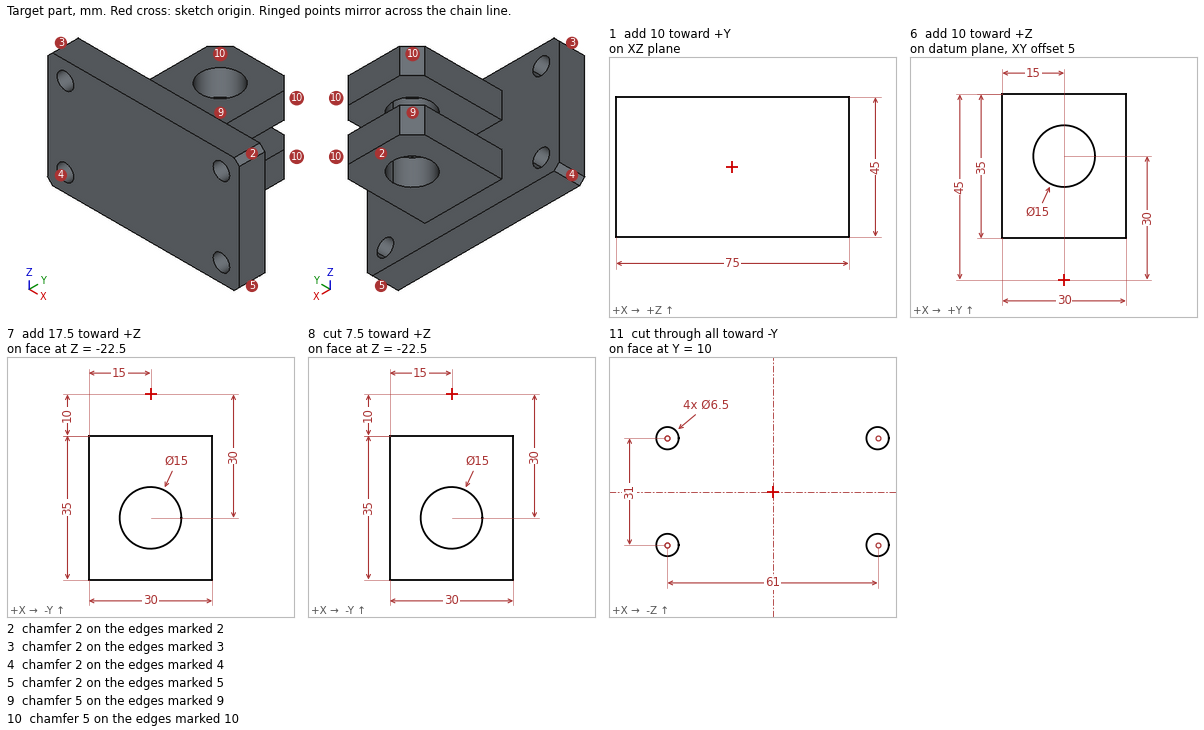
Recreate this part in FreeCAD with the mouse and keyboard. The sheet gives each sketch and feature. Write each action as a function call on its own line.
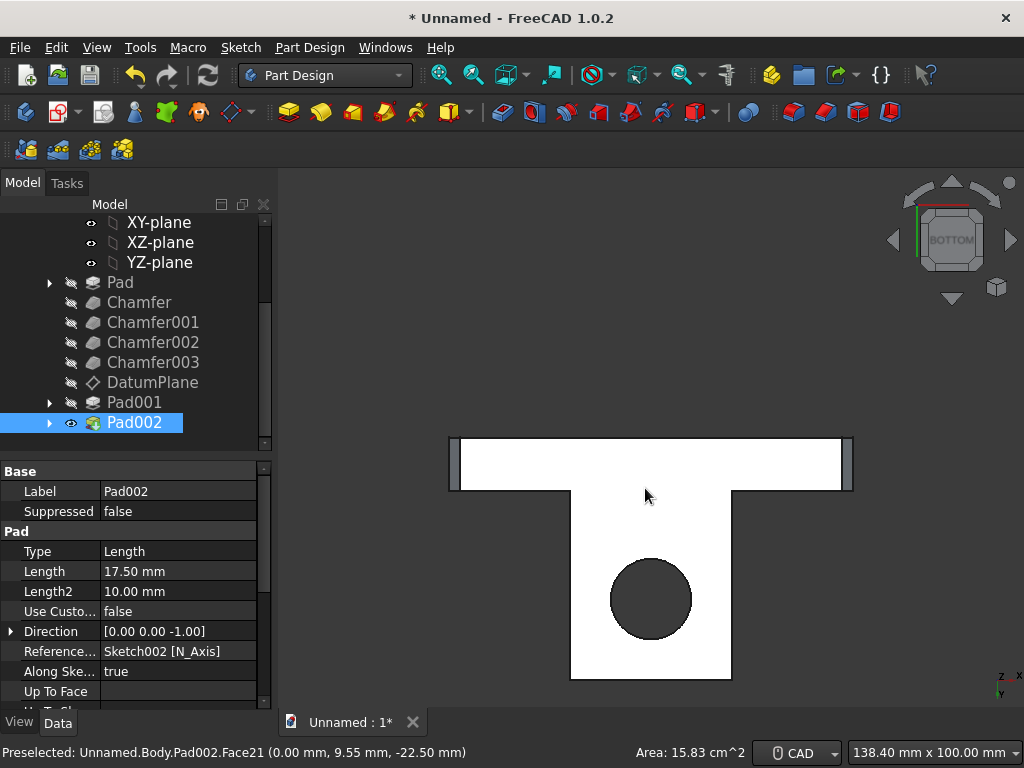
click(58, 112)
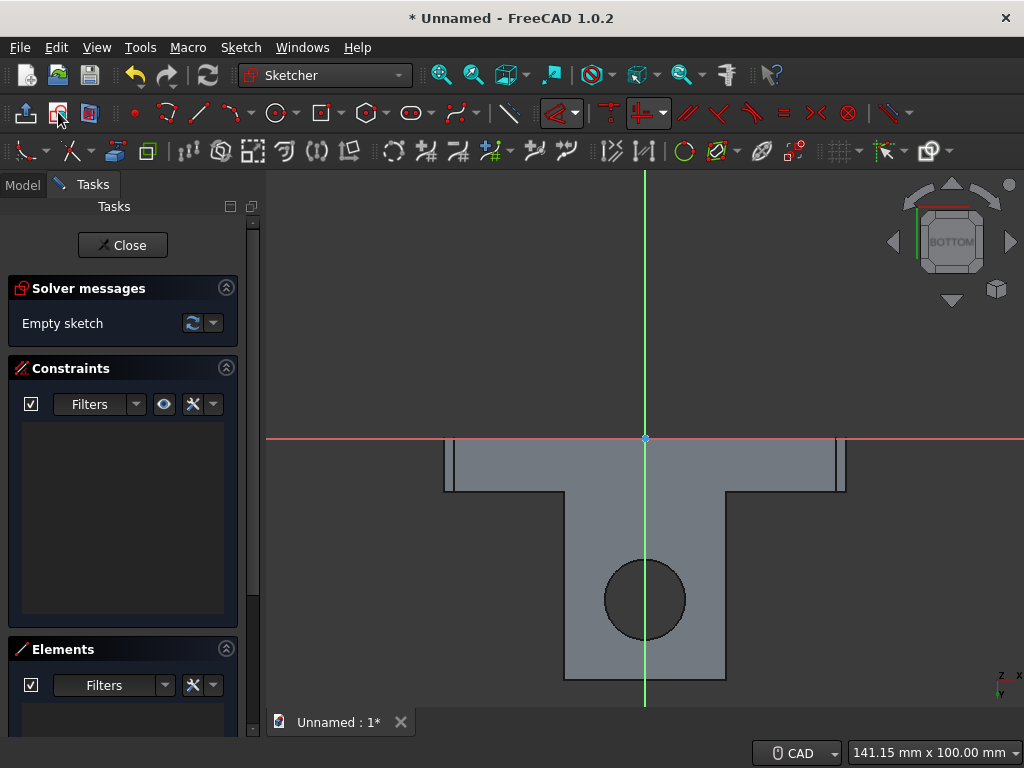
scroll(294, 198, down, 1)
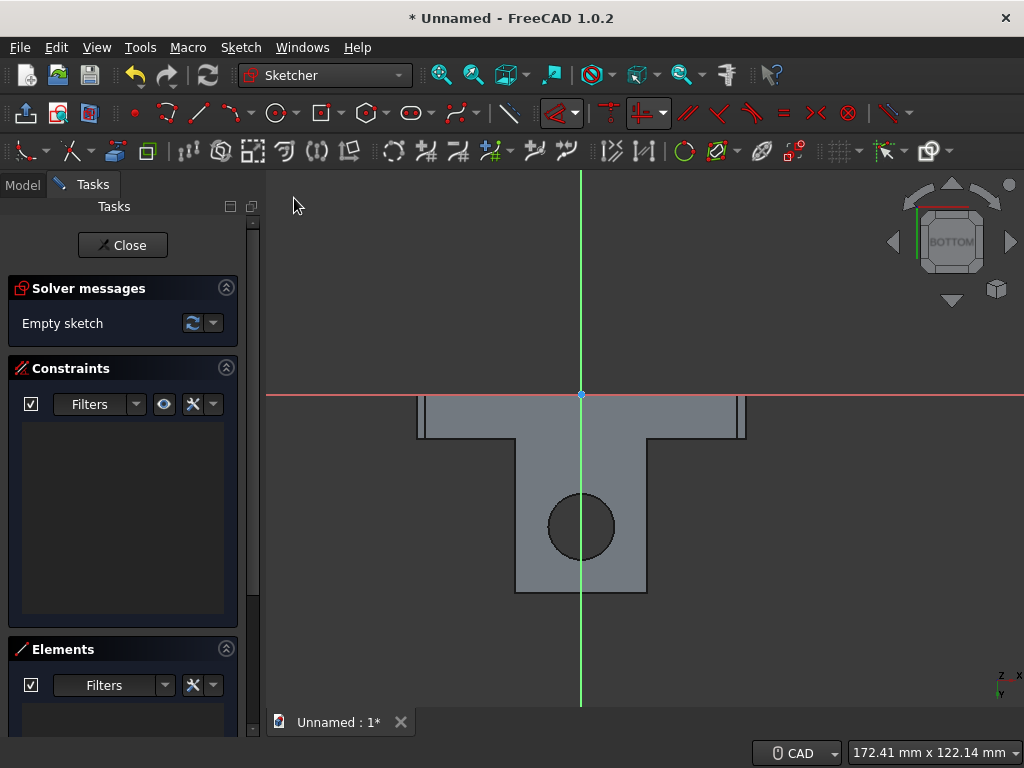
scroll(587, 561, up, 3)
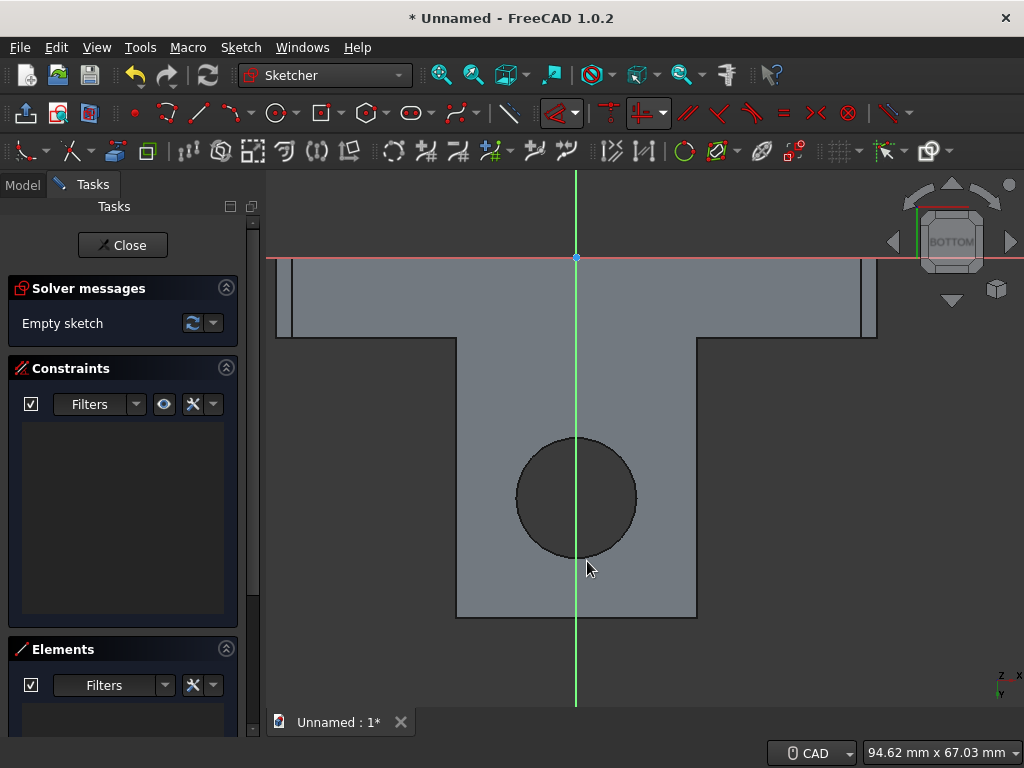
key(g)
key(r)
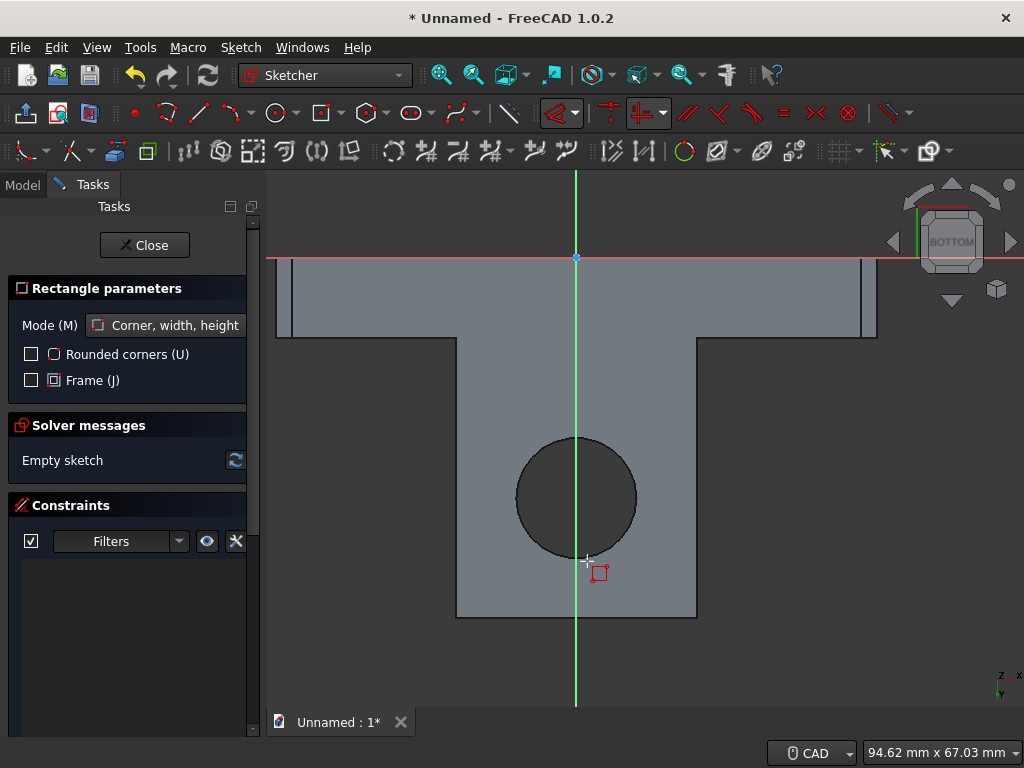
click(456, 338)
click(697, 618)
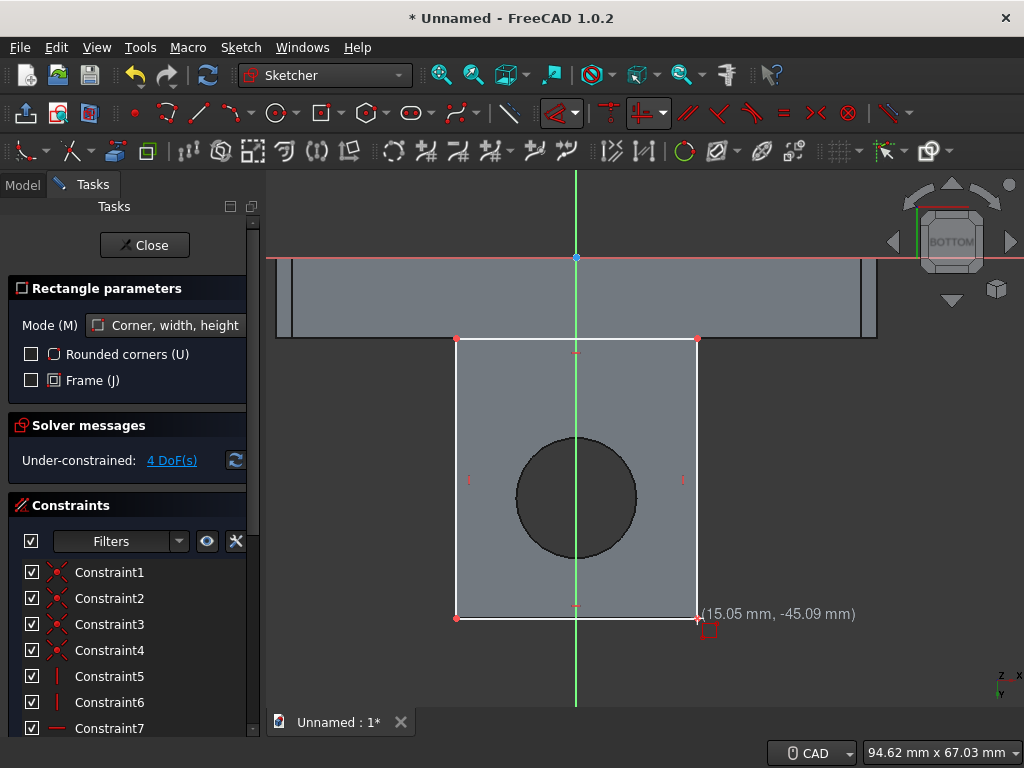
key(g)
key(c)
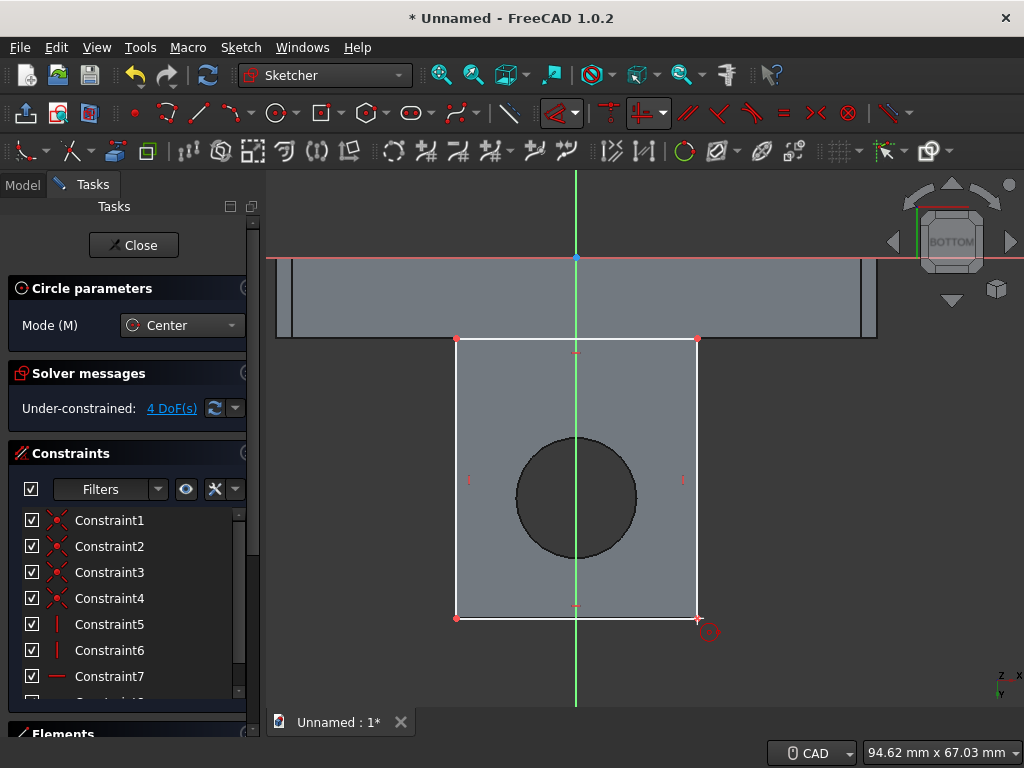
click(576, 498)
click(619, 456)
key(Escape)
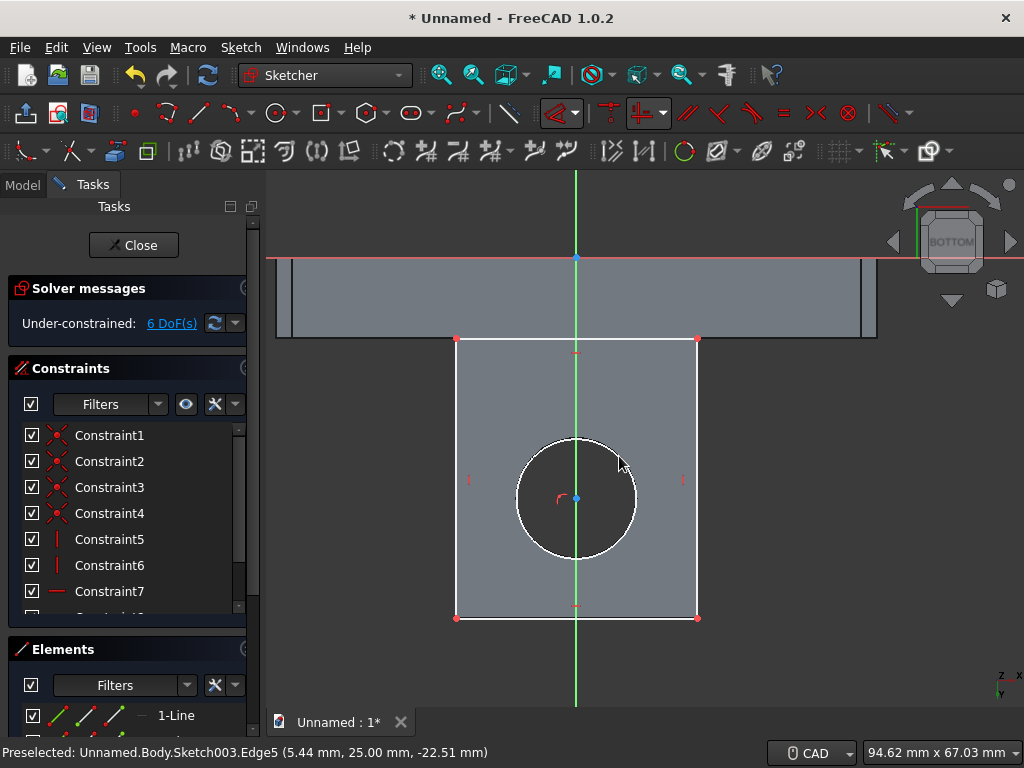
key(d)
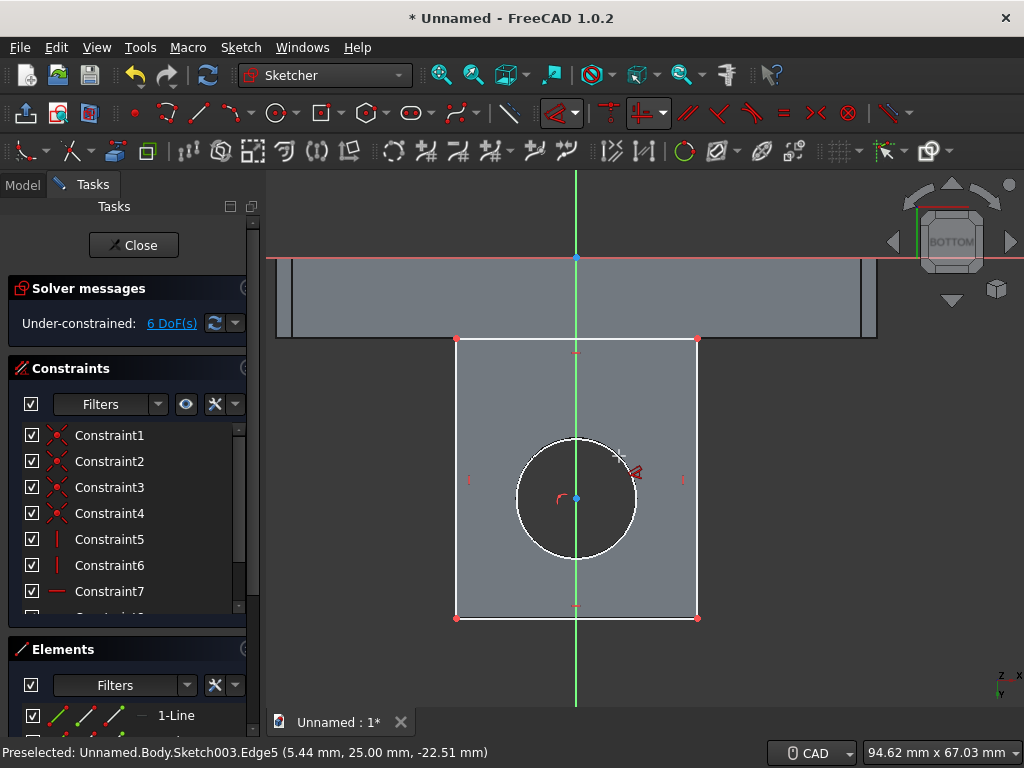
click(619, 457)
click(642, 435)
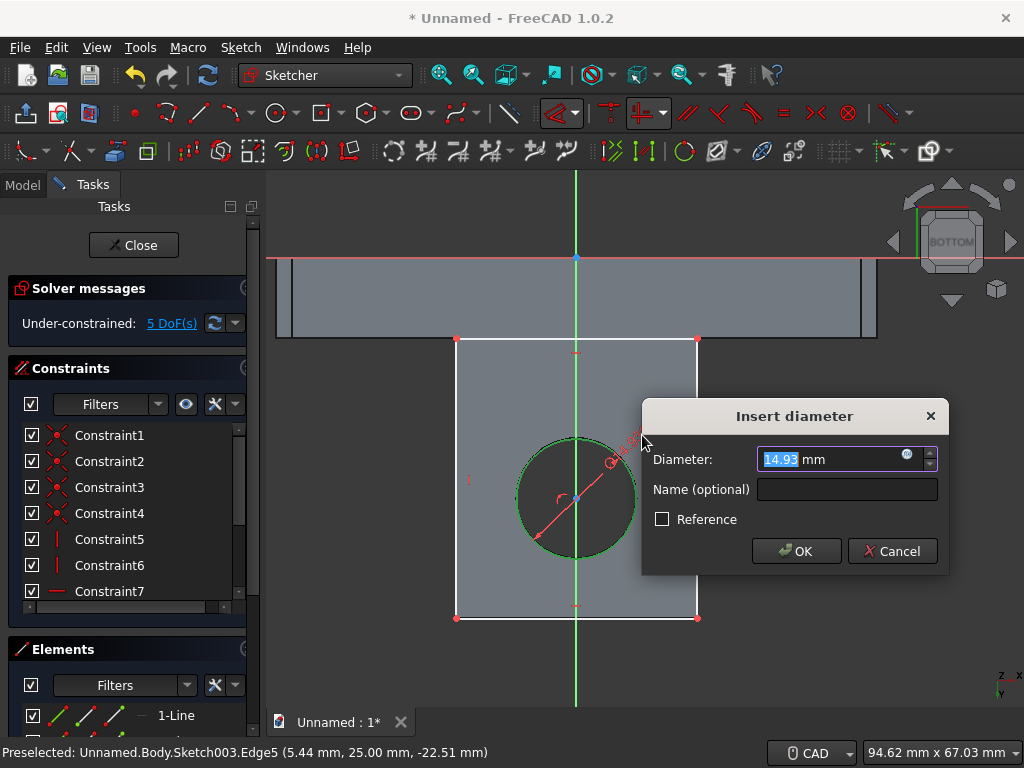
text(15)
key(Return)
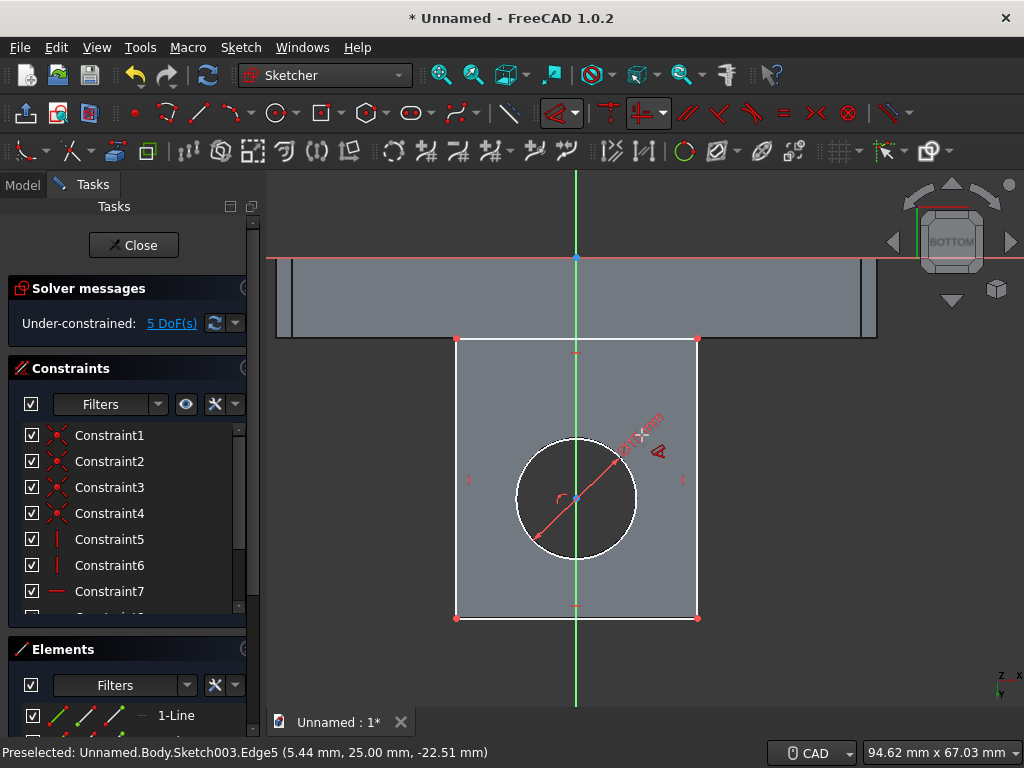
click(456, 423)
click(422, 479)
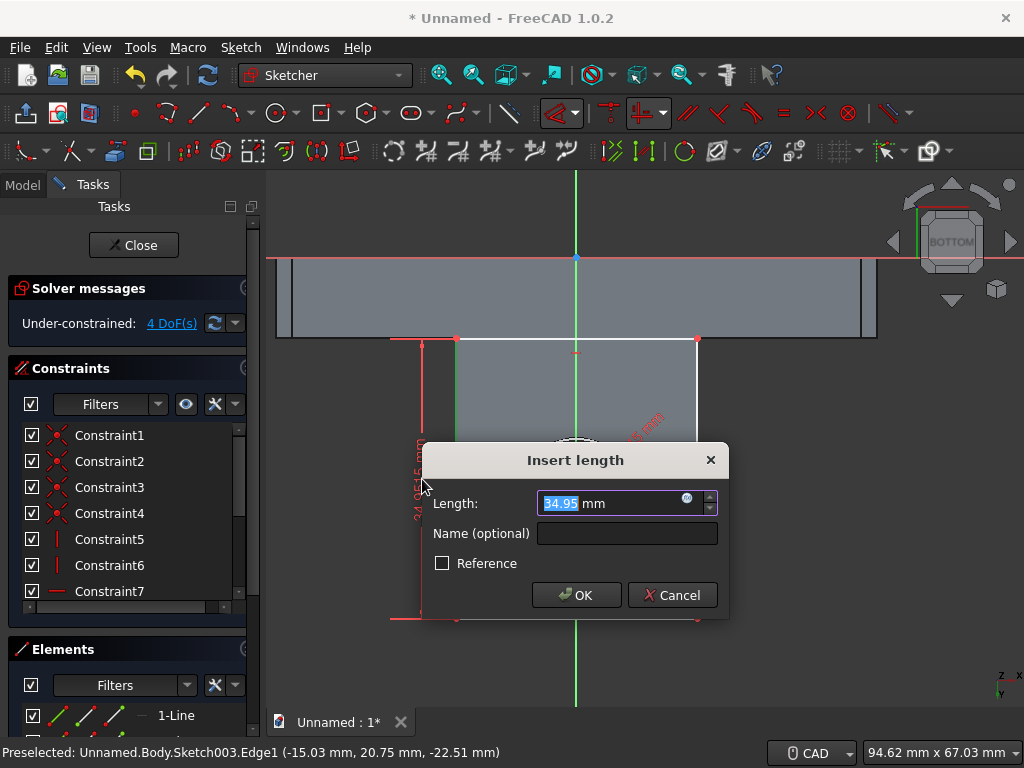
text(35)
key(Return)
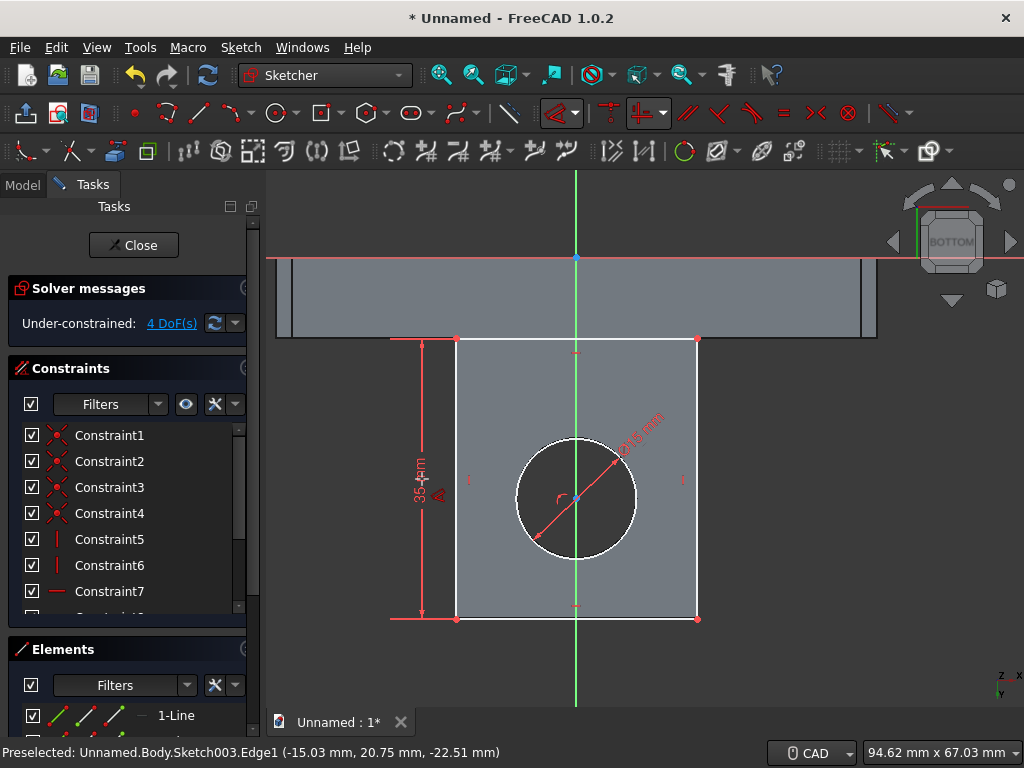
click(528, 619)
click(521, 653)